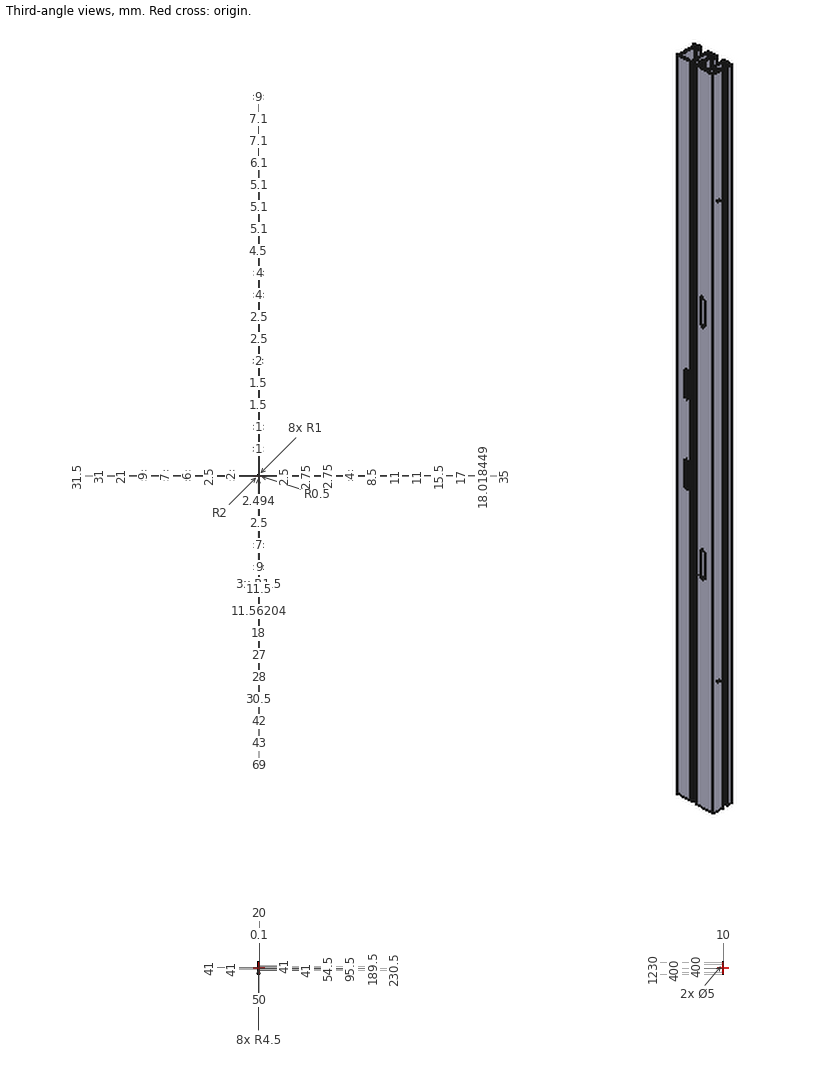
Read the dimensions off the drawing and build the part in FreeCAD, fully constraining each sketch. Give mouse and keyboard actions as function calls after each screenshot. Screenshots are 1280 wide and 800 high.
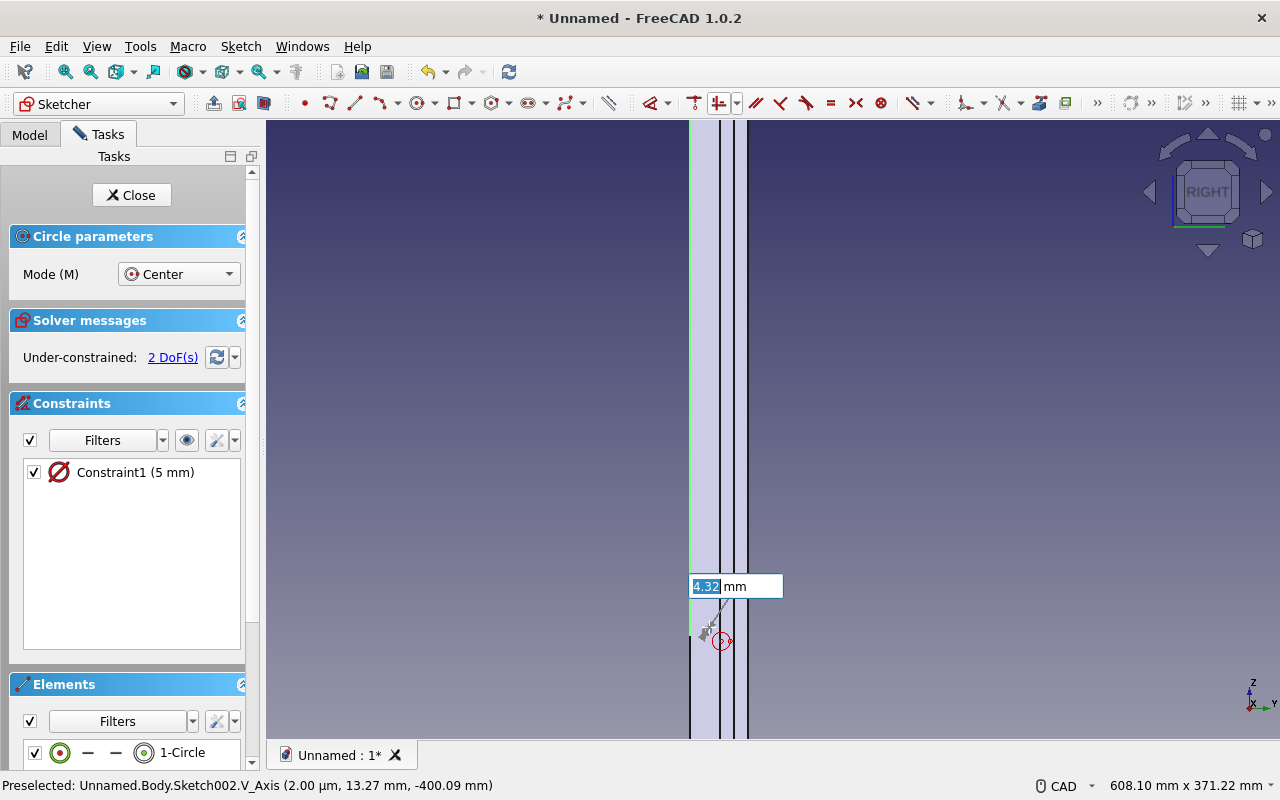
text(5)
key(Return)
key(Escape)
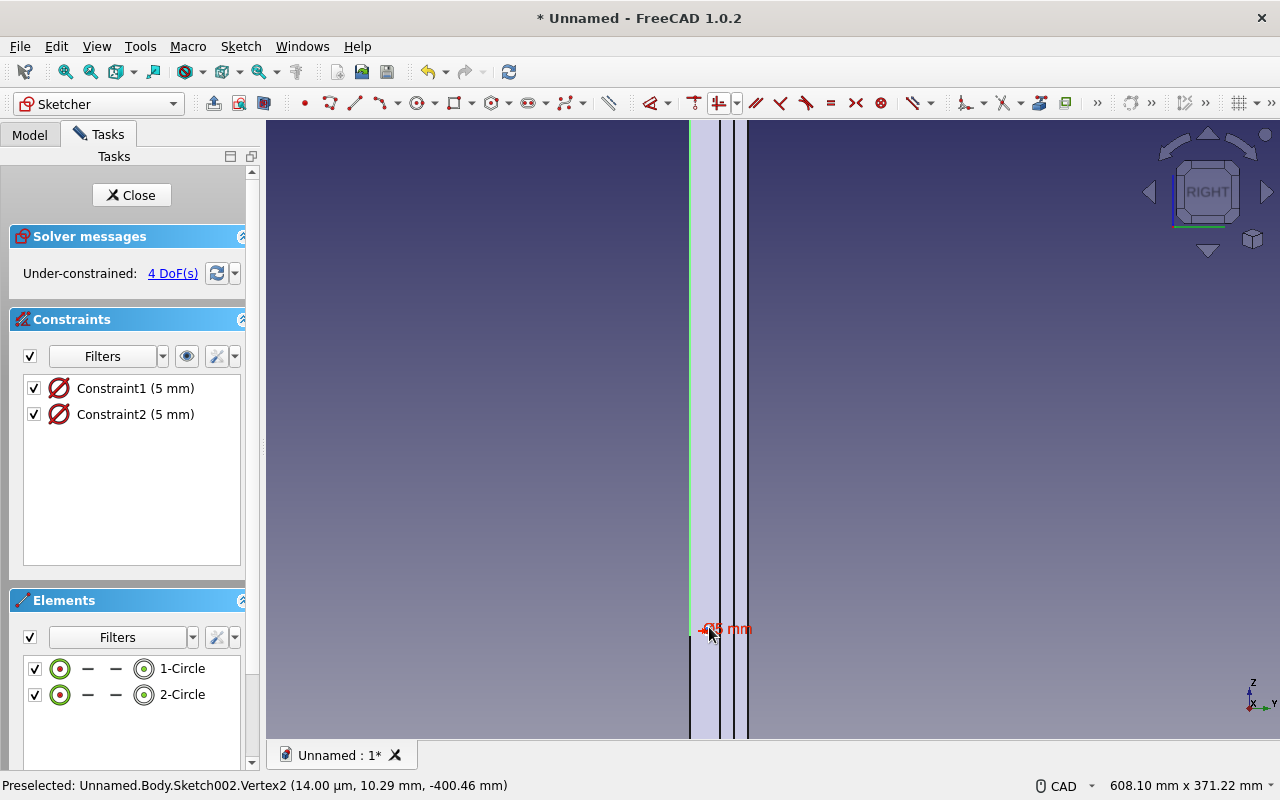
scroll(706, 630, down, 6)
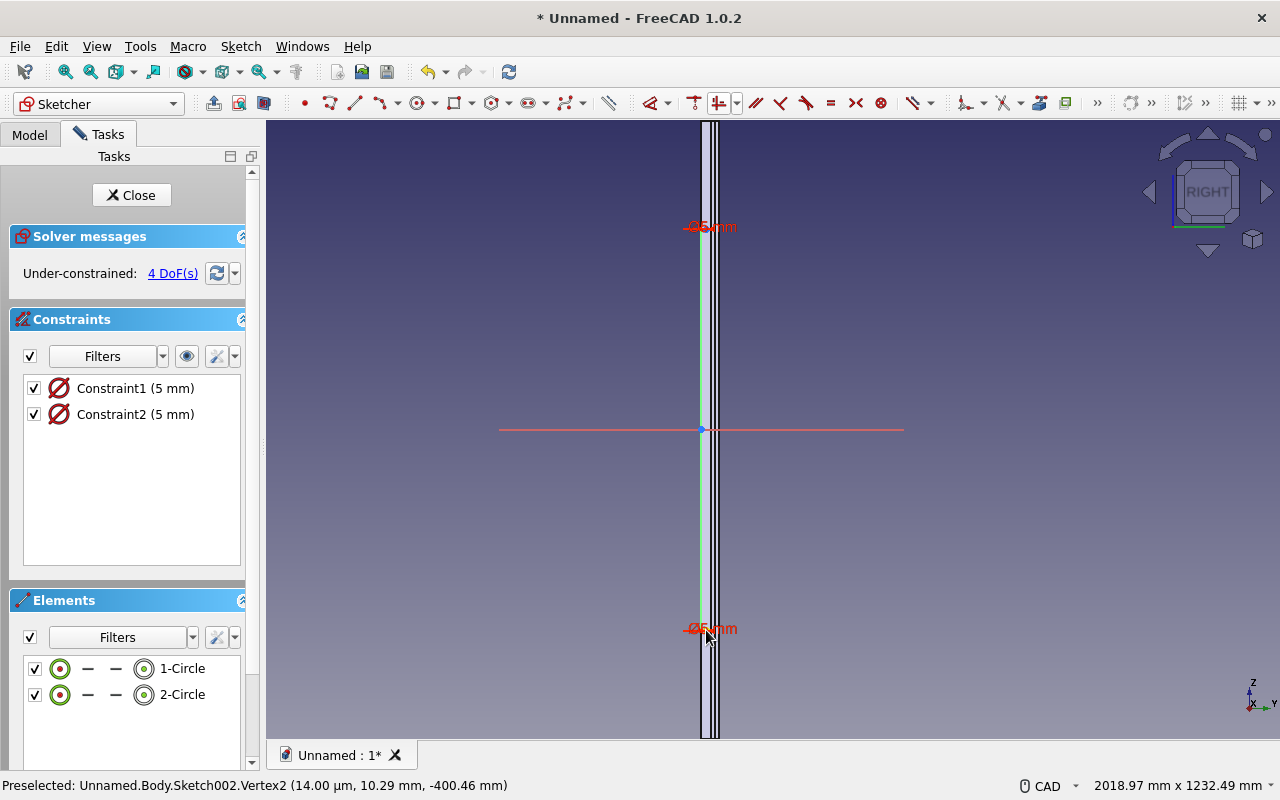
click(707, 229)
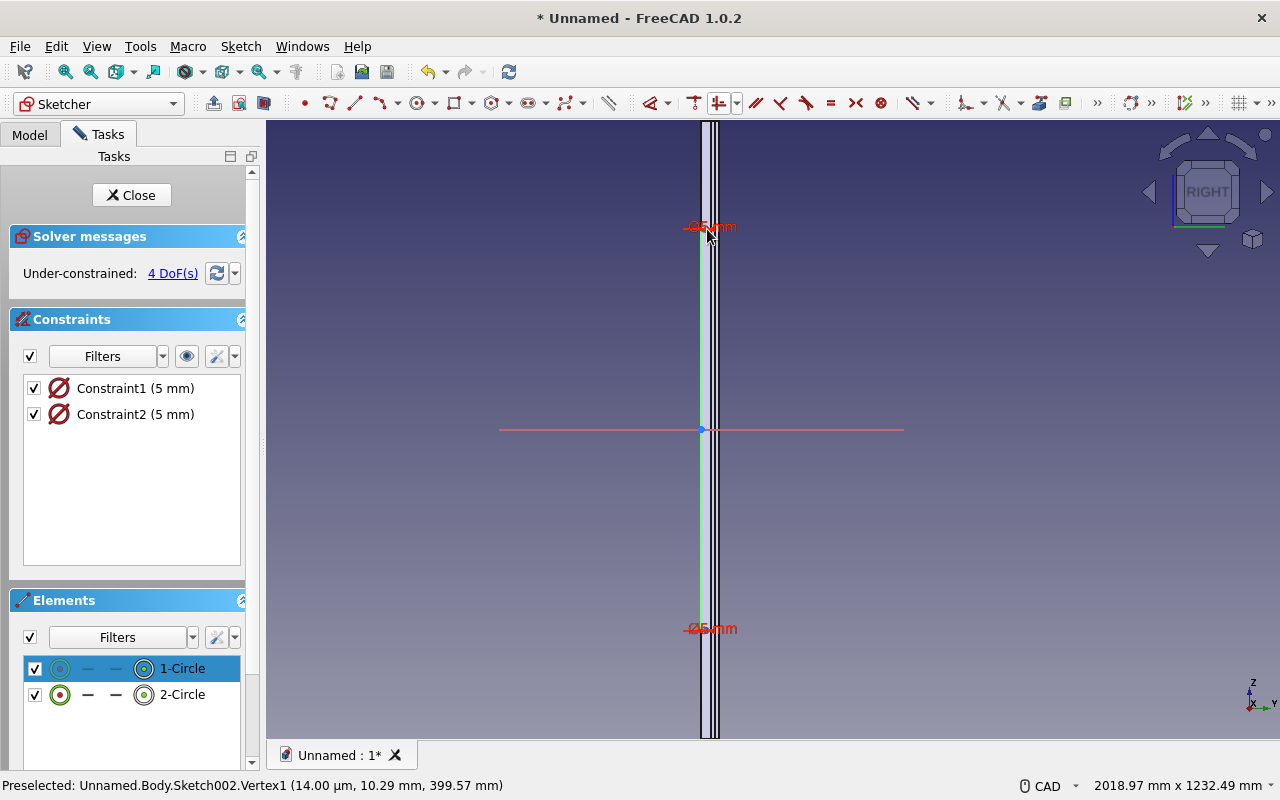
click(707, 631)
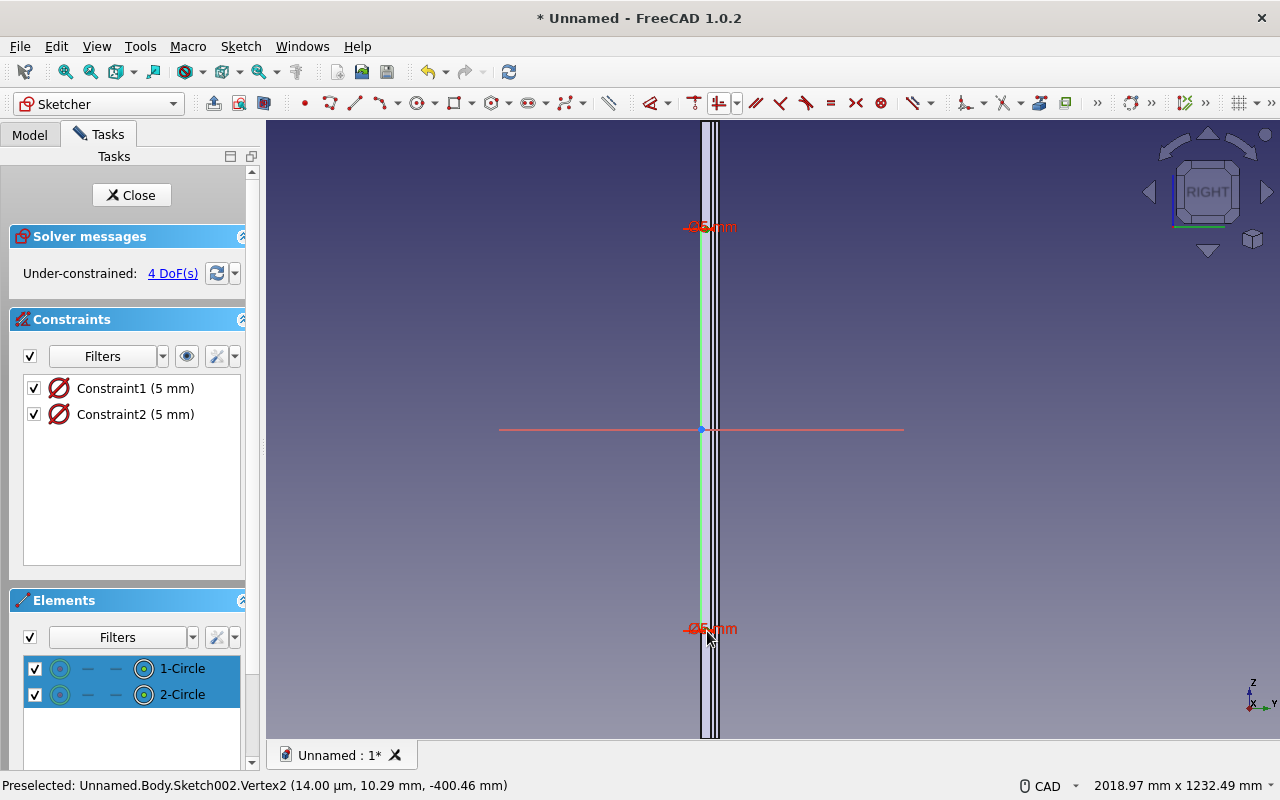
click(736, 104)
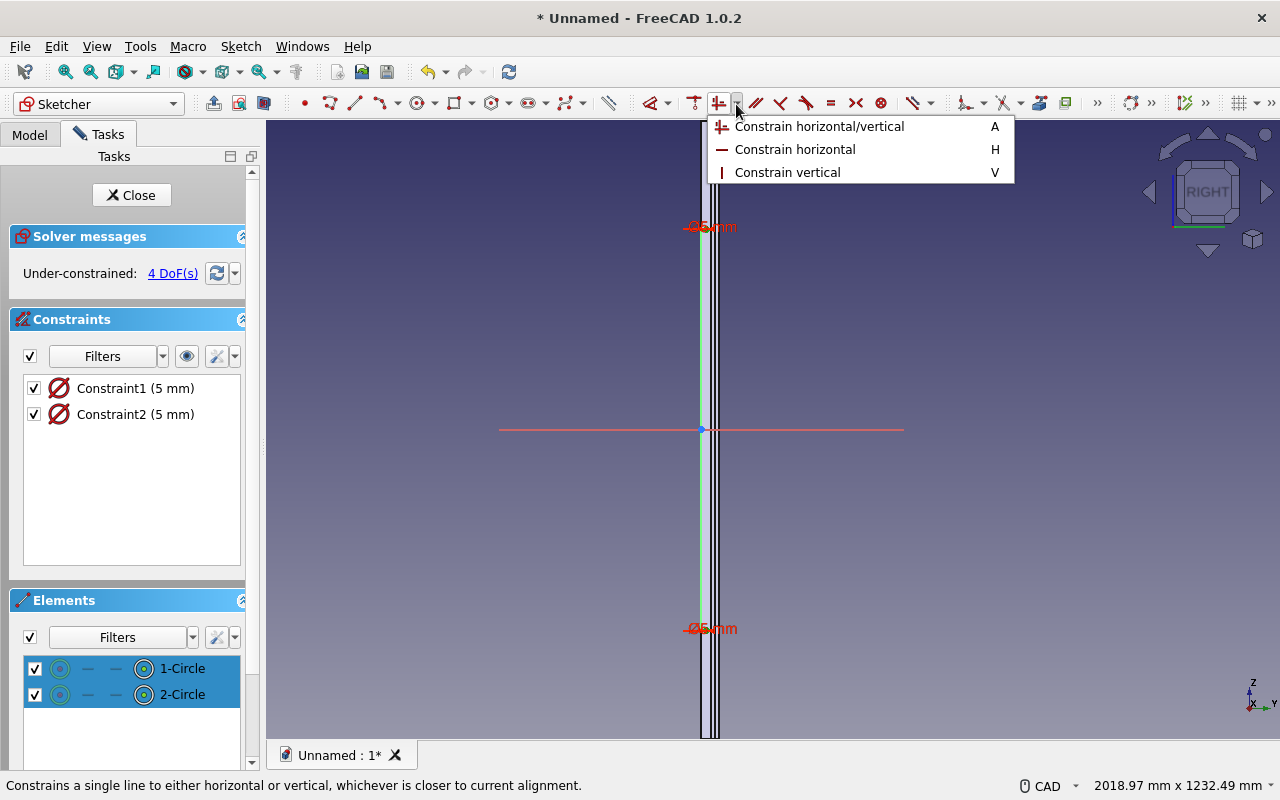
click(861, 172)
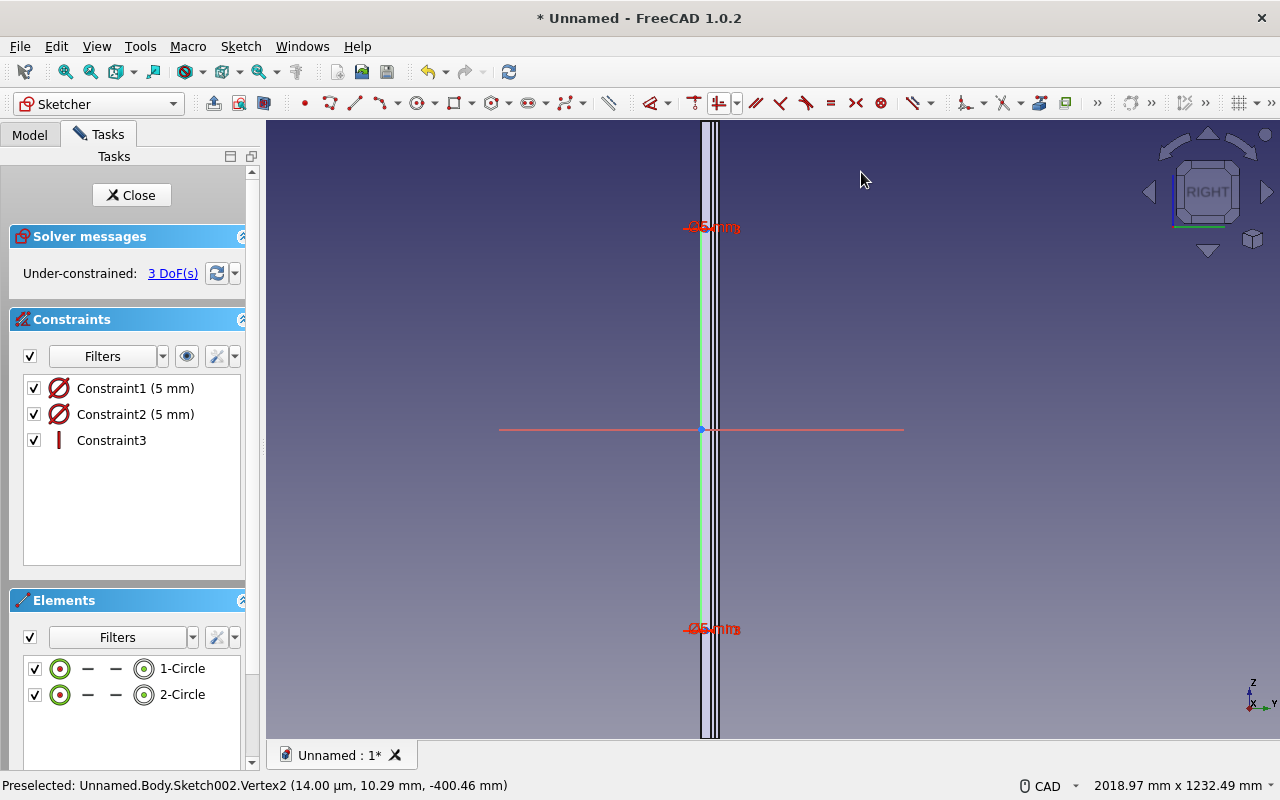
click(650, 104)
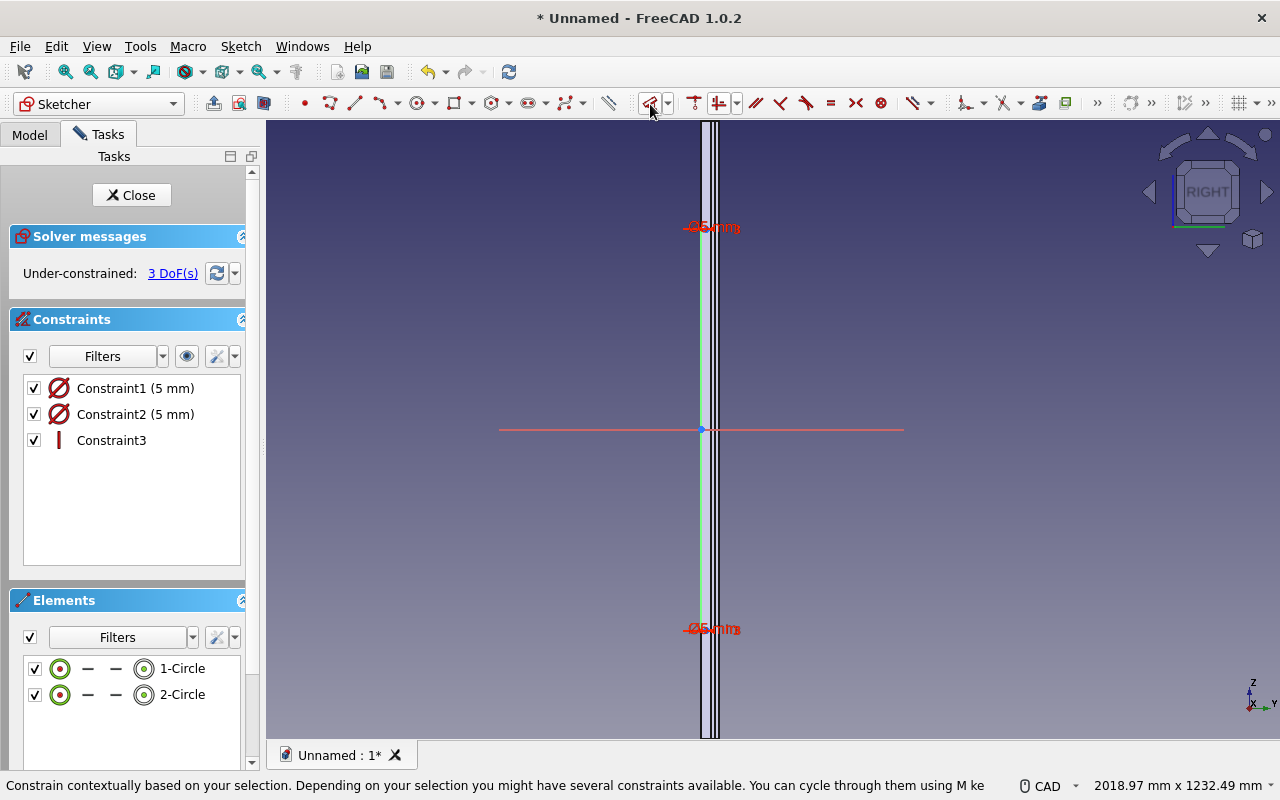
scroll(707, 229, up, 11)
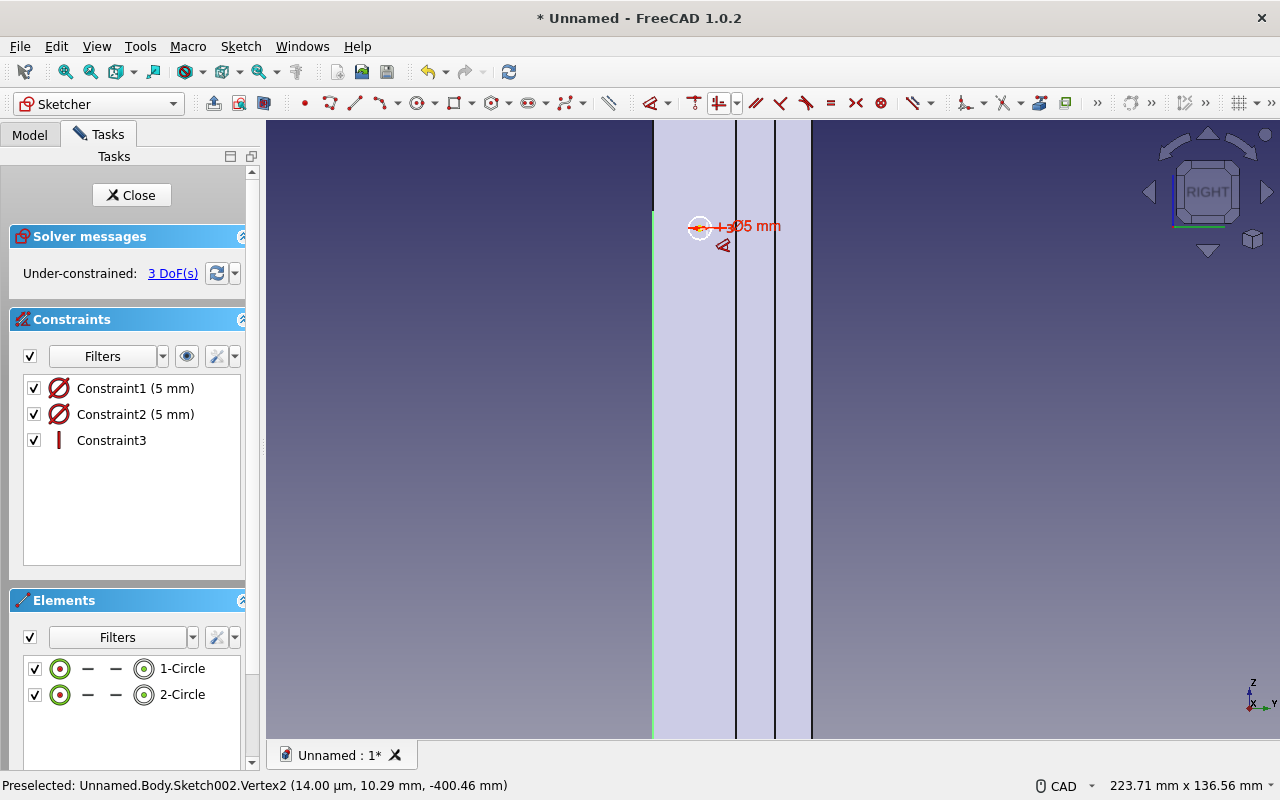
click(700, 228)
click(677, 194)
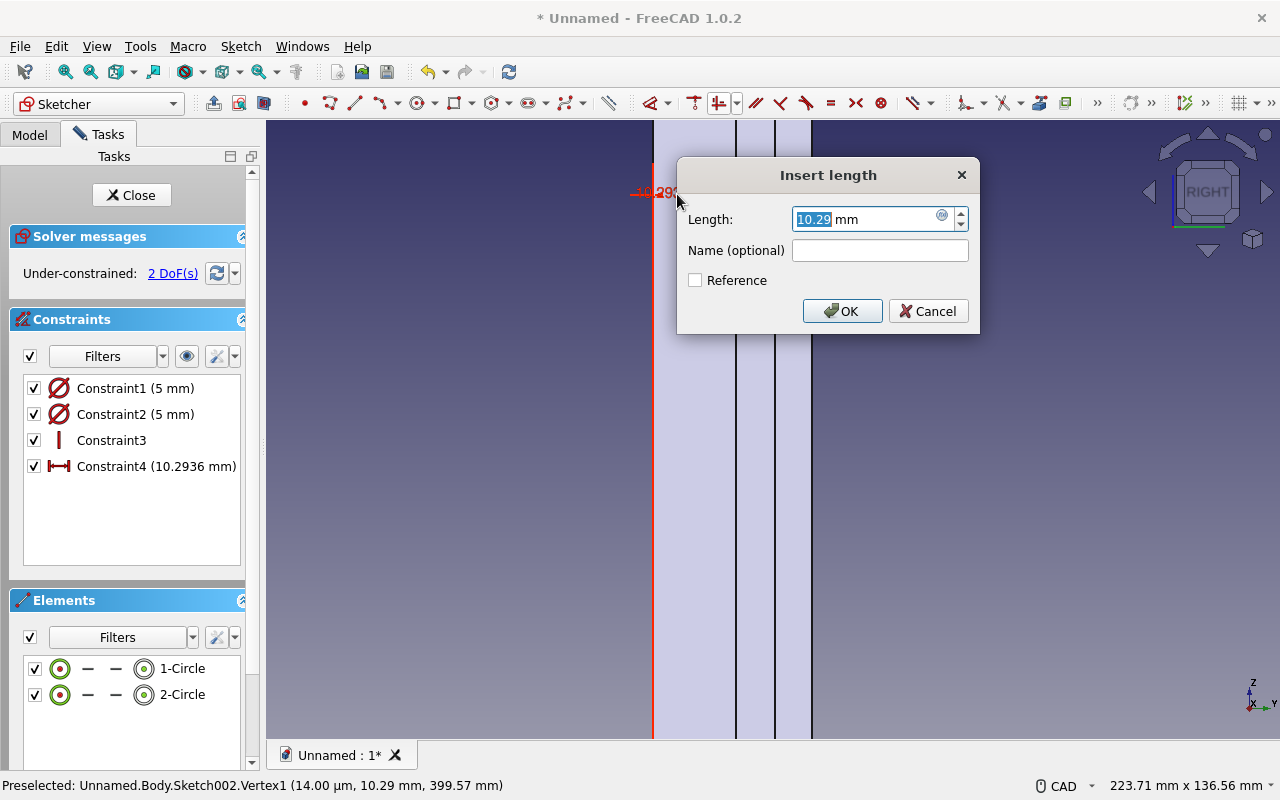
text(10)
key(Return)